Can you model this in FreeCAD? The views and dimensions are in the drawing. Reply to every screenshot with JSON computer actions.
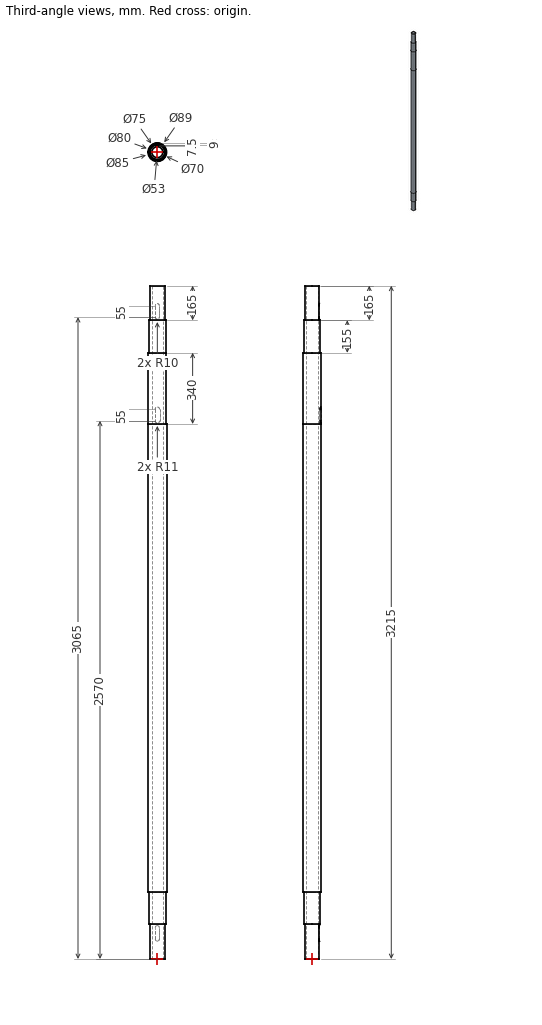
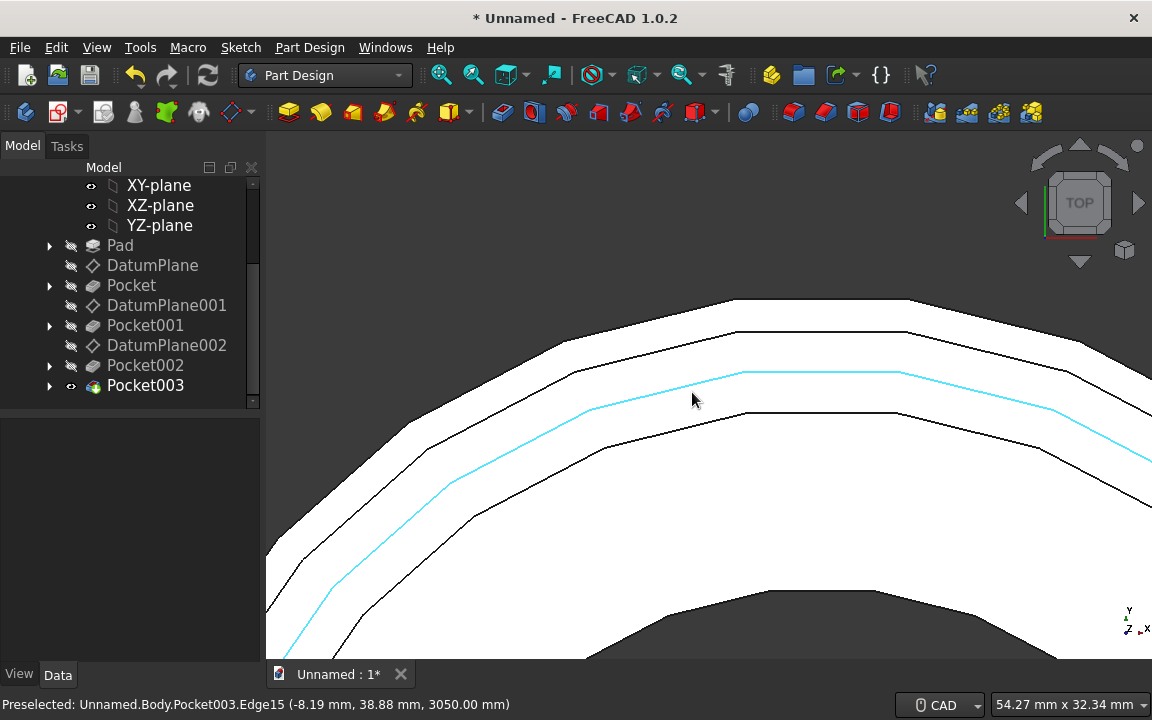
{"action": "left_click", "coordinate": [690, 394]}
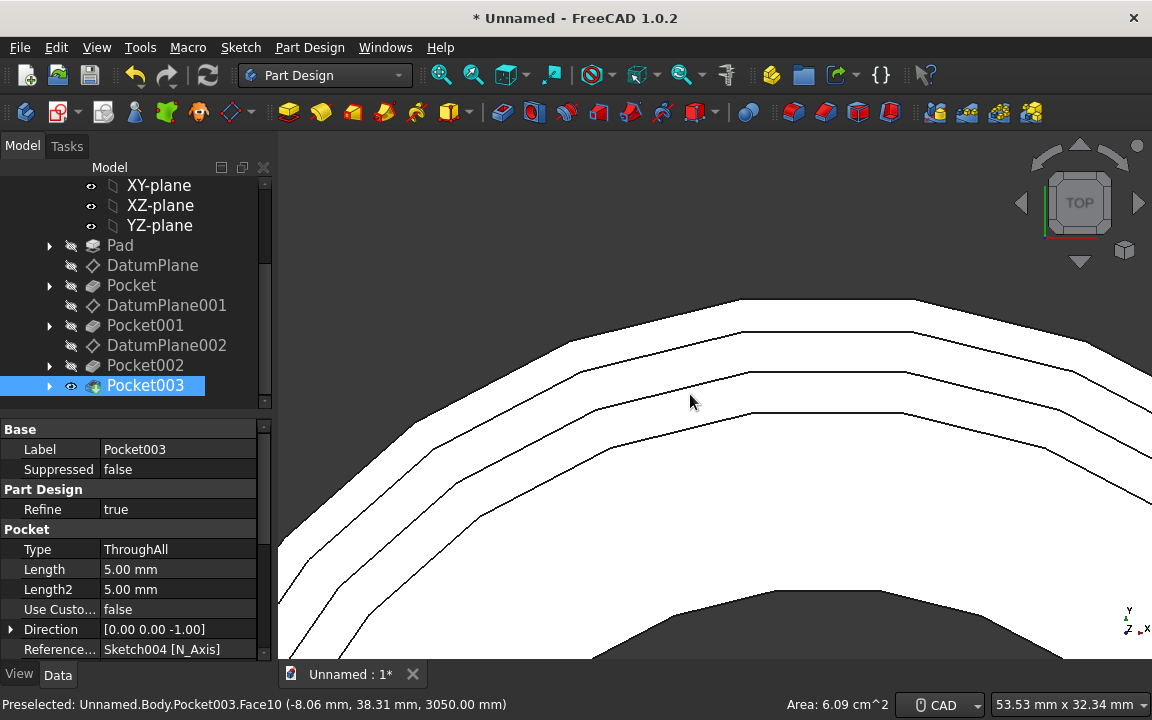
{"action": "left_click", "coordinate": [58, 112]}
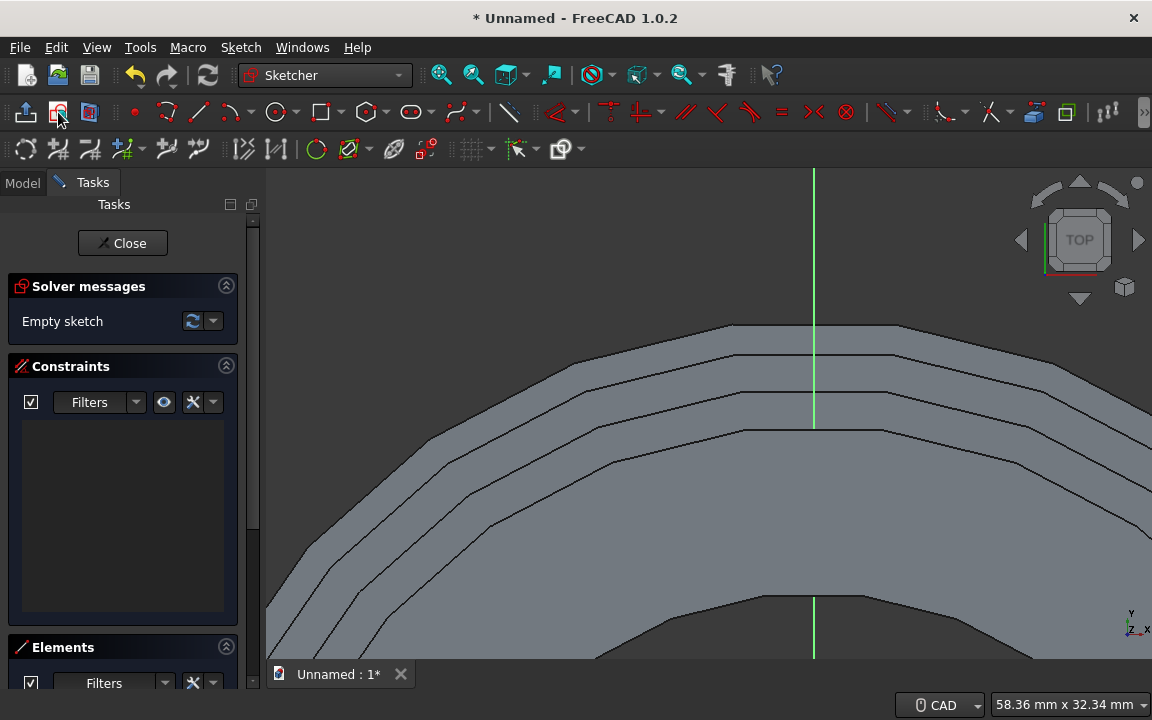
{"action": "scroll", "coordinate": [584, 223], "scroll_direction": "down", "scroll_amount": 7}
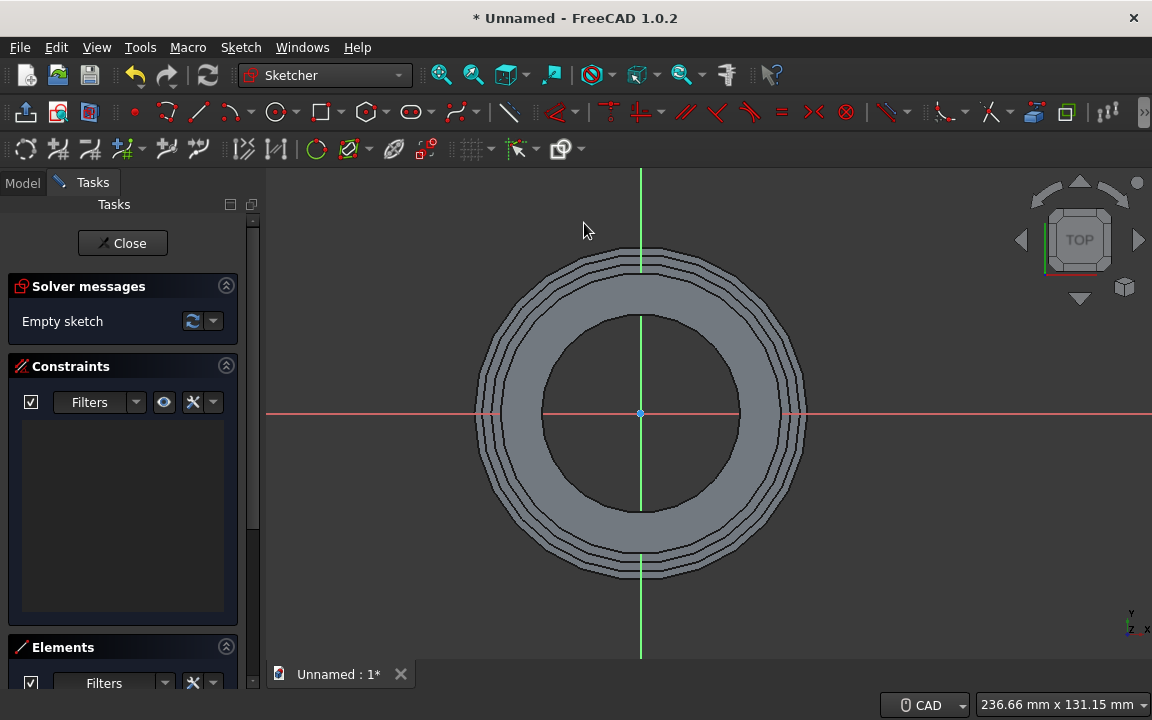
{"action": "left_click", "coordinate": [276, 112]}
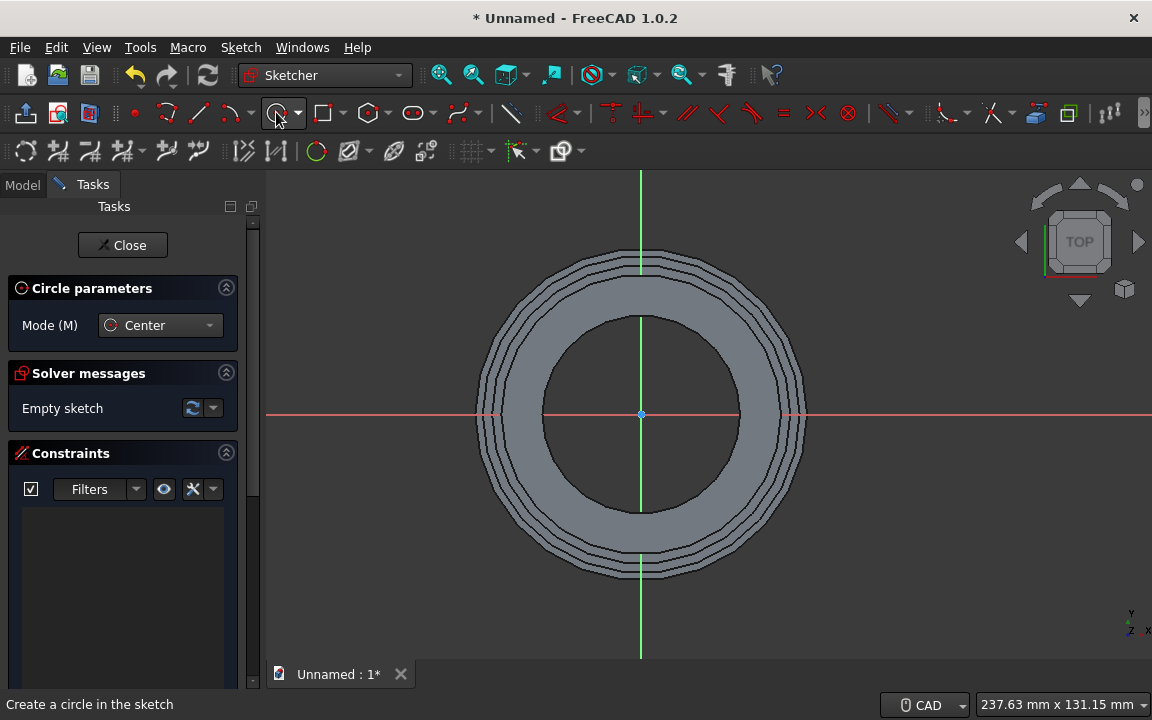
{"action": "left_click", "coordinate": [641, 415]}
{"action": "mouse_move", "coordinate": [740, 316]}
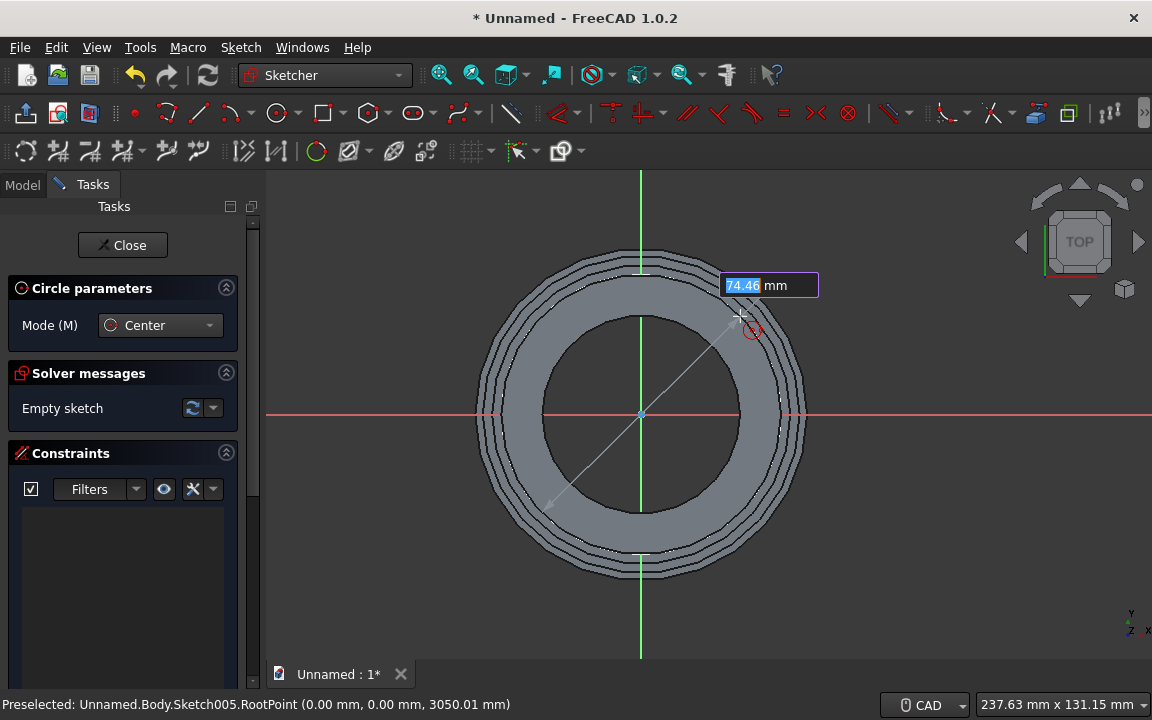
{"action": "type", "text": "75"}
{"action": "key", "text": "Return"}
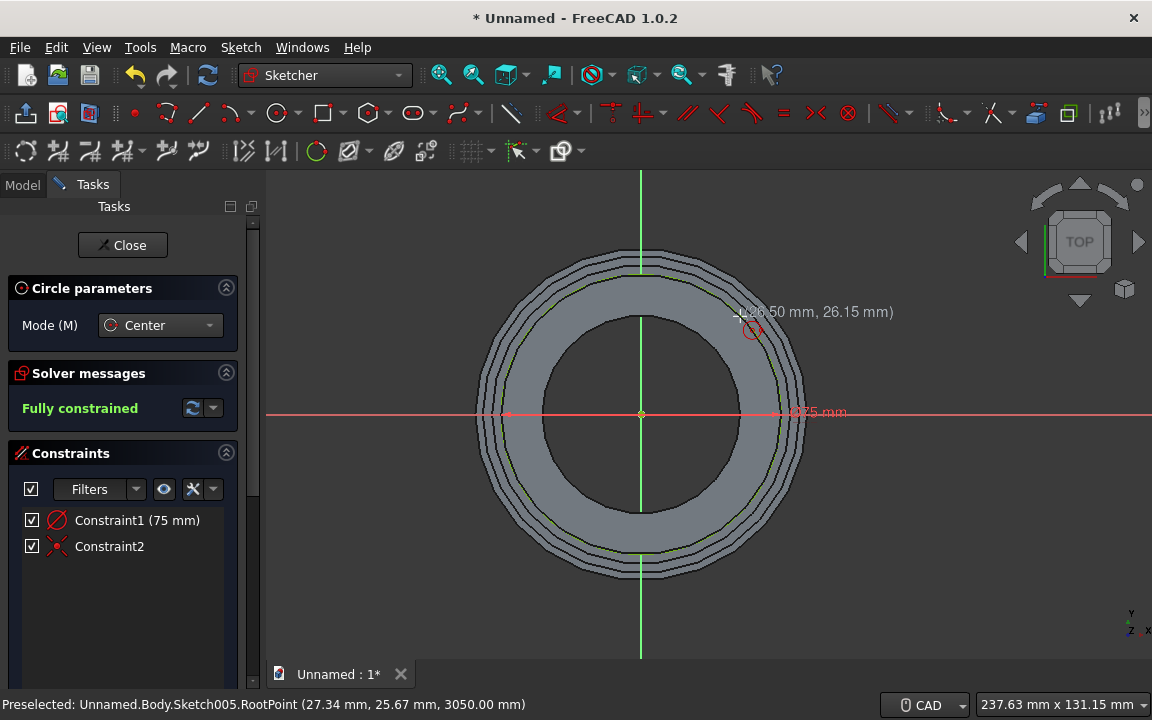
{"action": "left_click", "coordinate": [641, 415]}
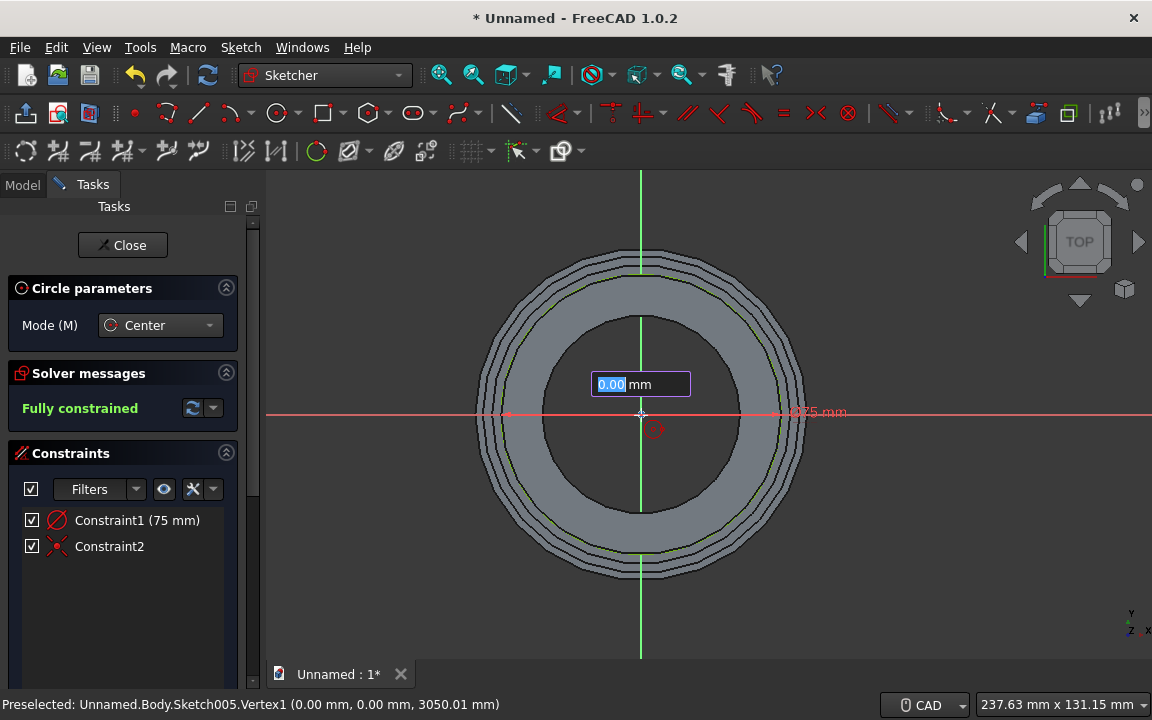
{"action": "scroll", "coordinate": [733, 322], "scroll_direction": "up", "scroll_amount": 3}
{"action": "mouse_move", "coordinate": [733, 322]}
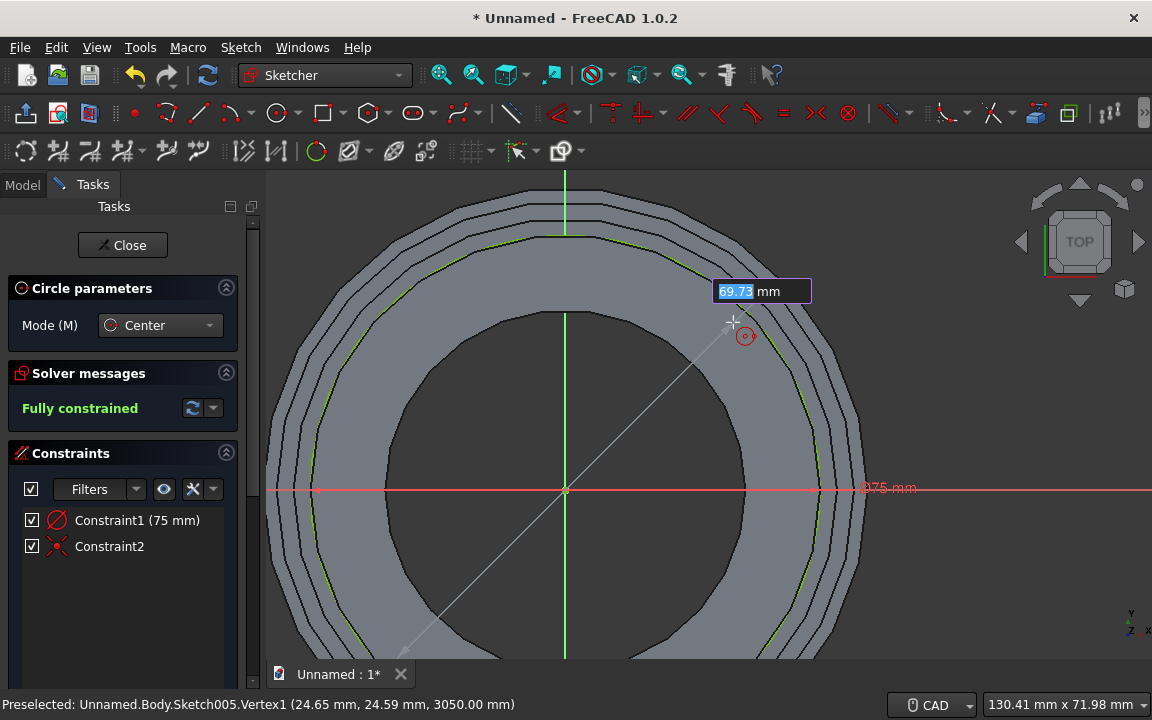
{"action": "type", "text": "70"}
{"action": "key", "text": "Return"}
{"action": "key", "text": "Escape"}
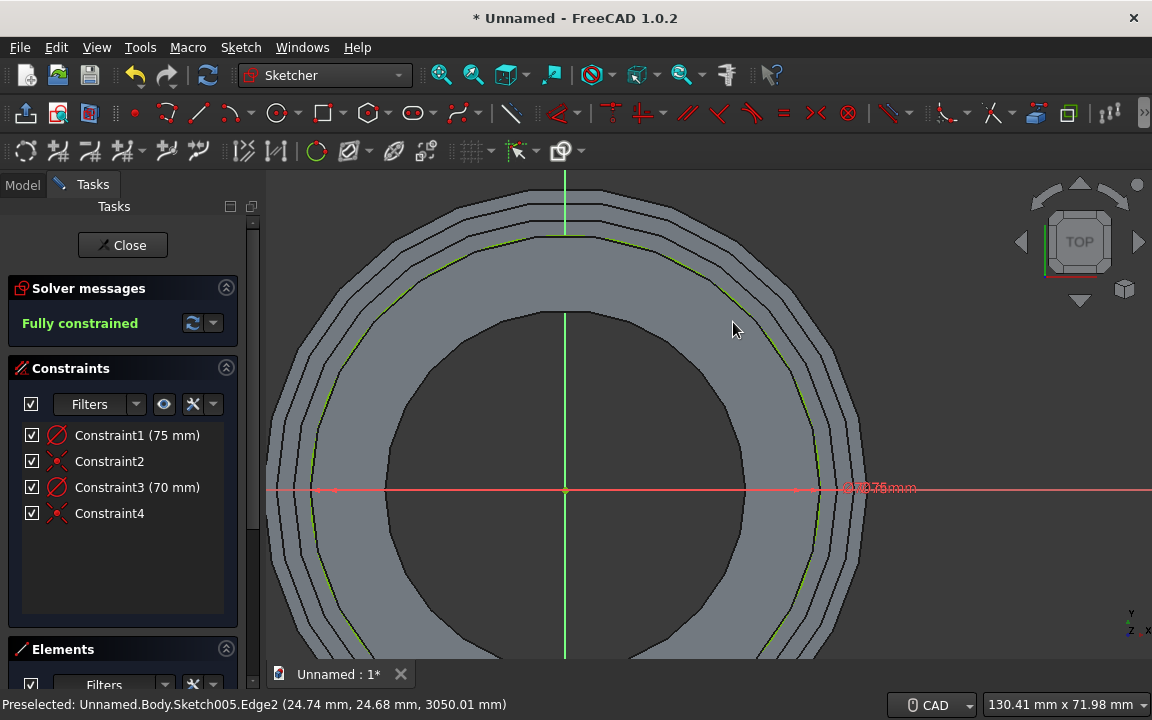
{"action": "left_click", "coordinate": [123, 245]}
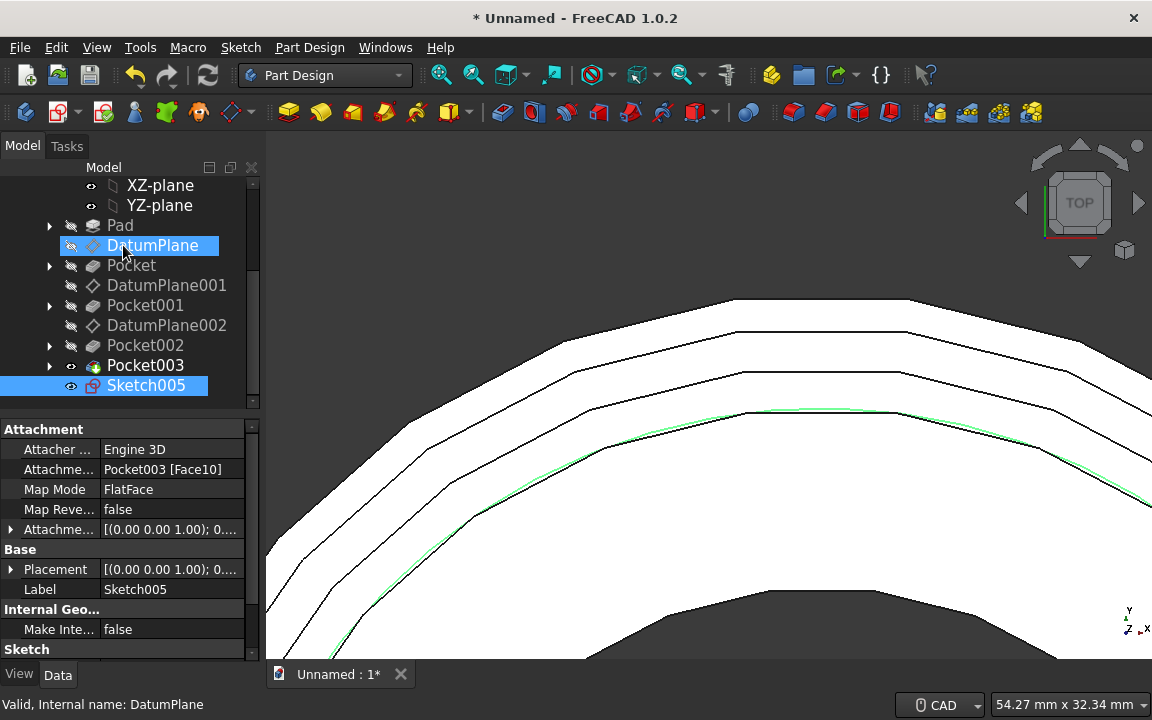
{"action": "left_click", "coordinate": [504, 112]}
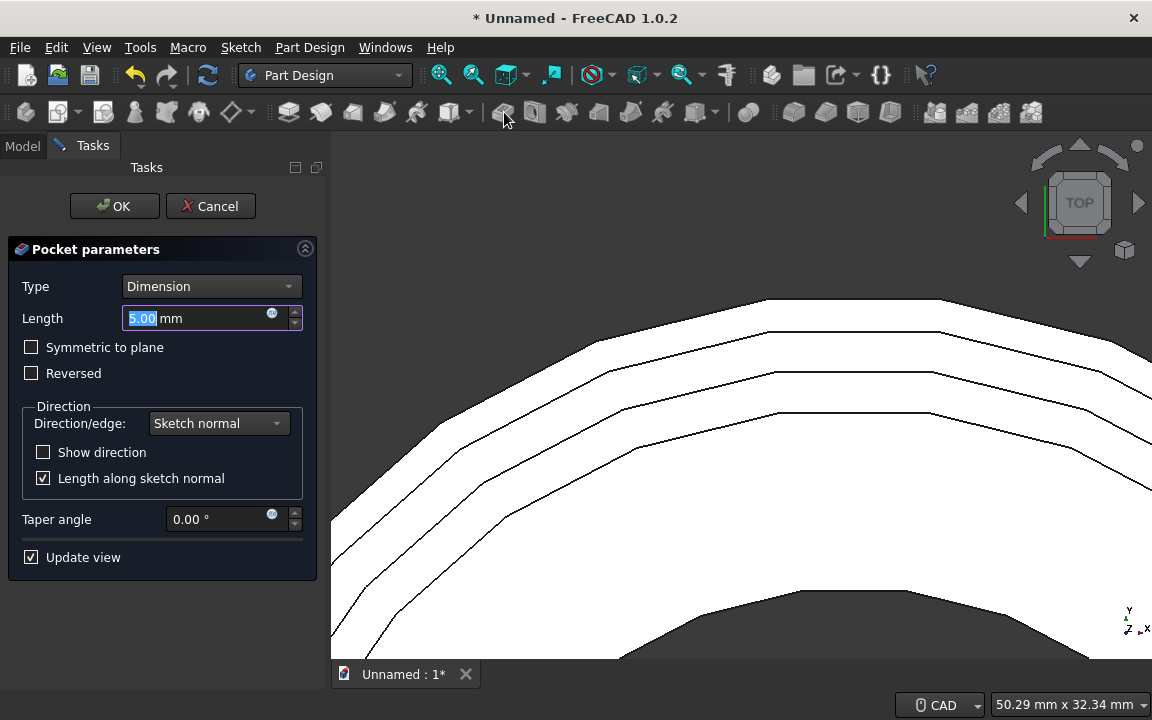
{"action": "type", "text": "165"}
{"action": "key", "text": "Tab"}